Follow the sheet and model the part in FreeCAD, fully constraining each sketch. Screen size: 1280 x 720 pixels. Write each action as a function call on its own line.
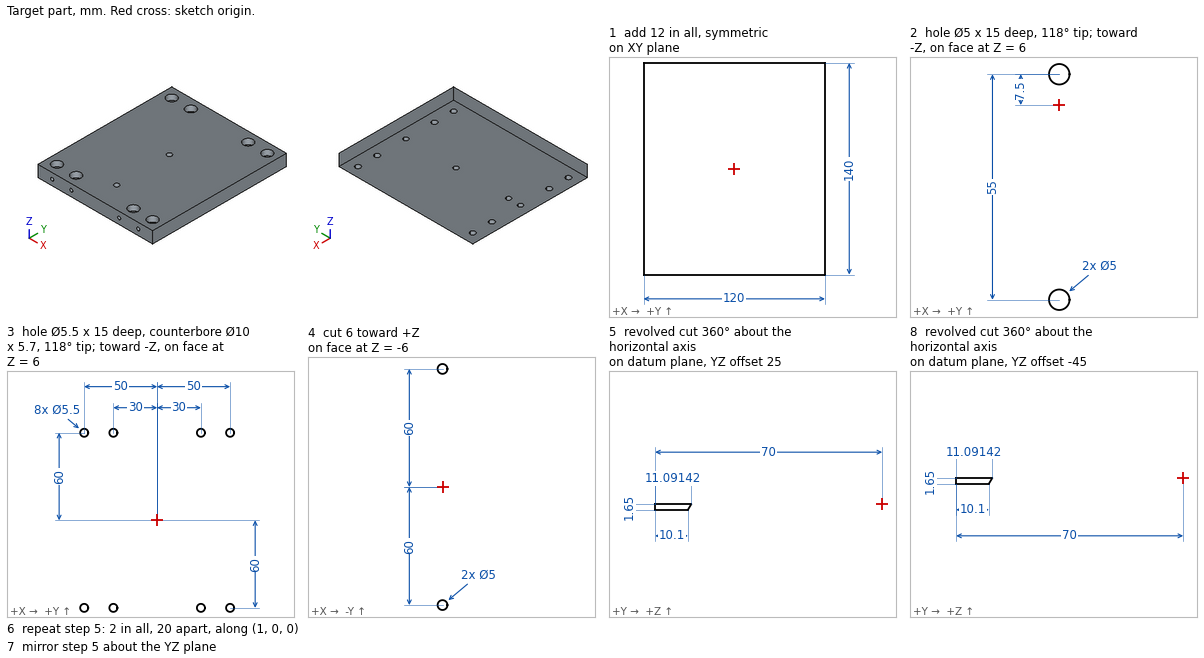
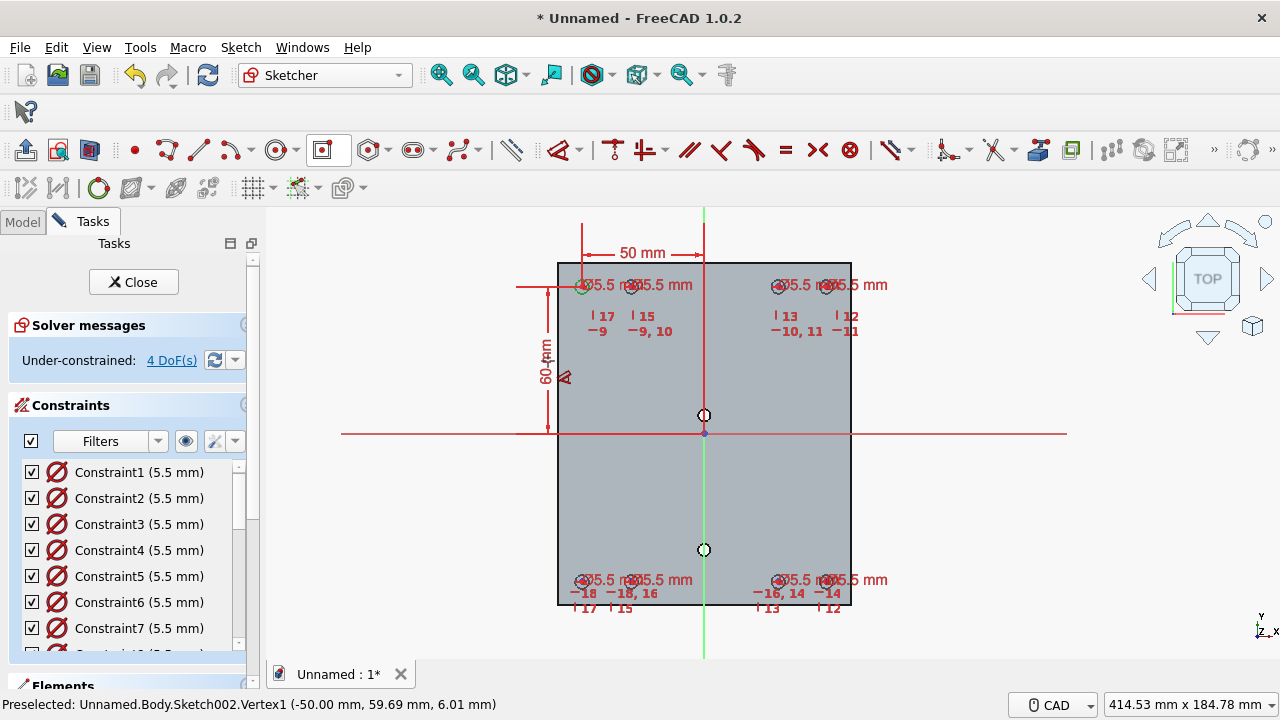
click(631, 287)
click(668, 468)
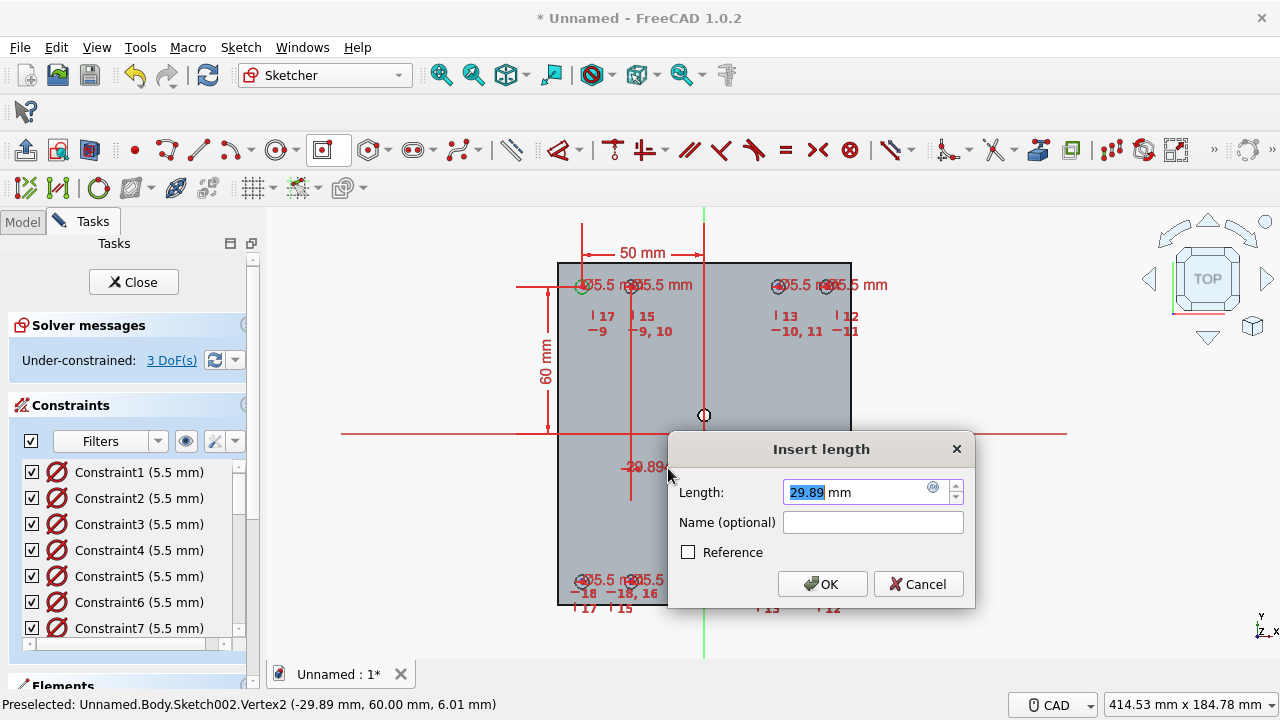
text(30)
key(Return)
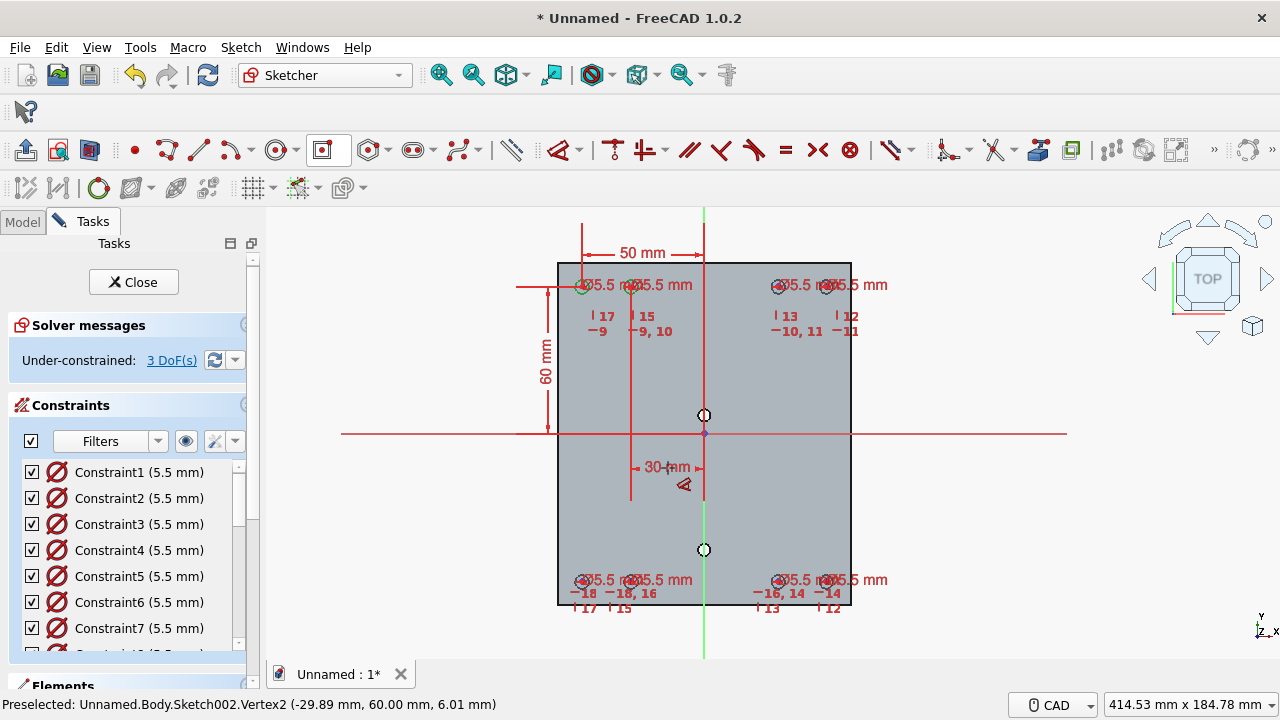
click(778, 287)
click(741, 253)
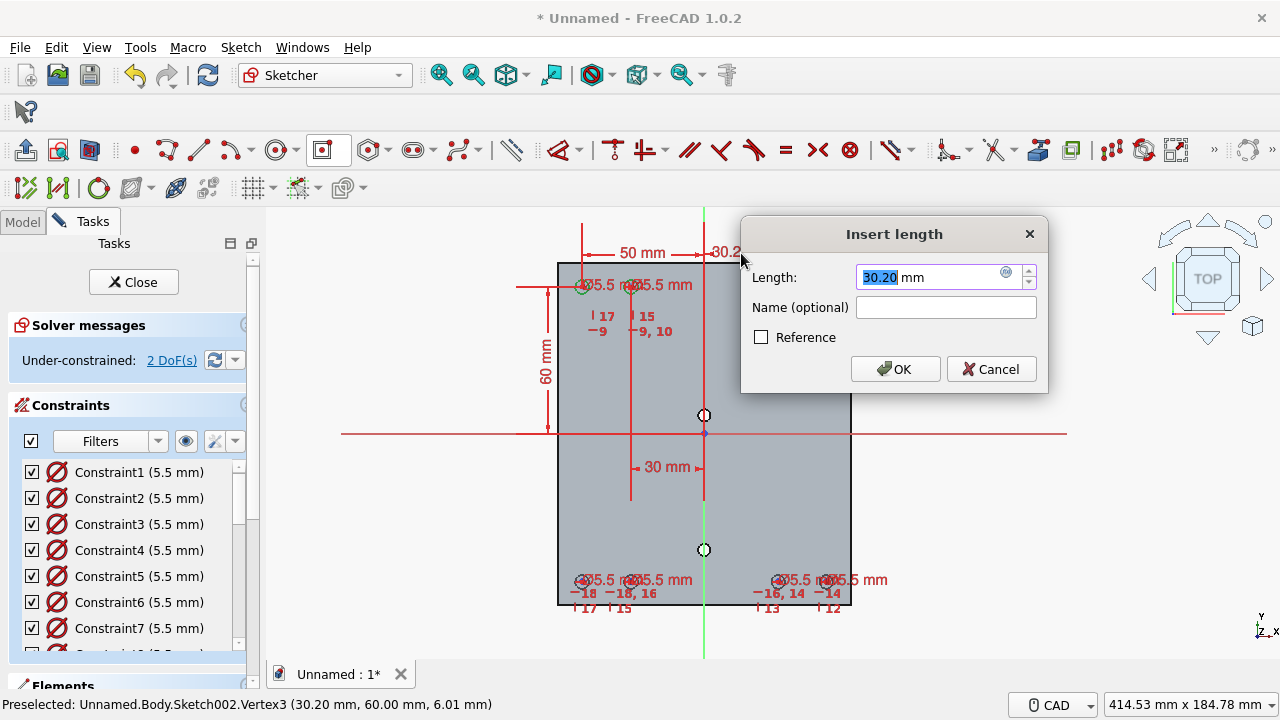
text(30)
key(Return)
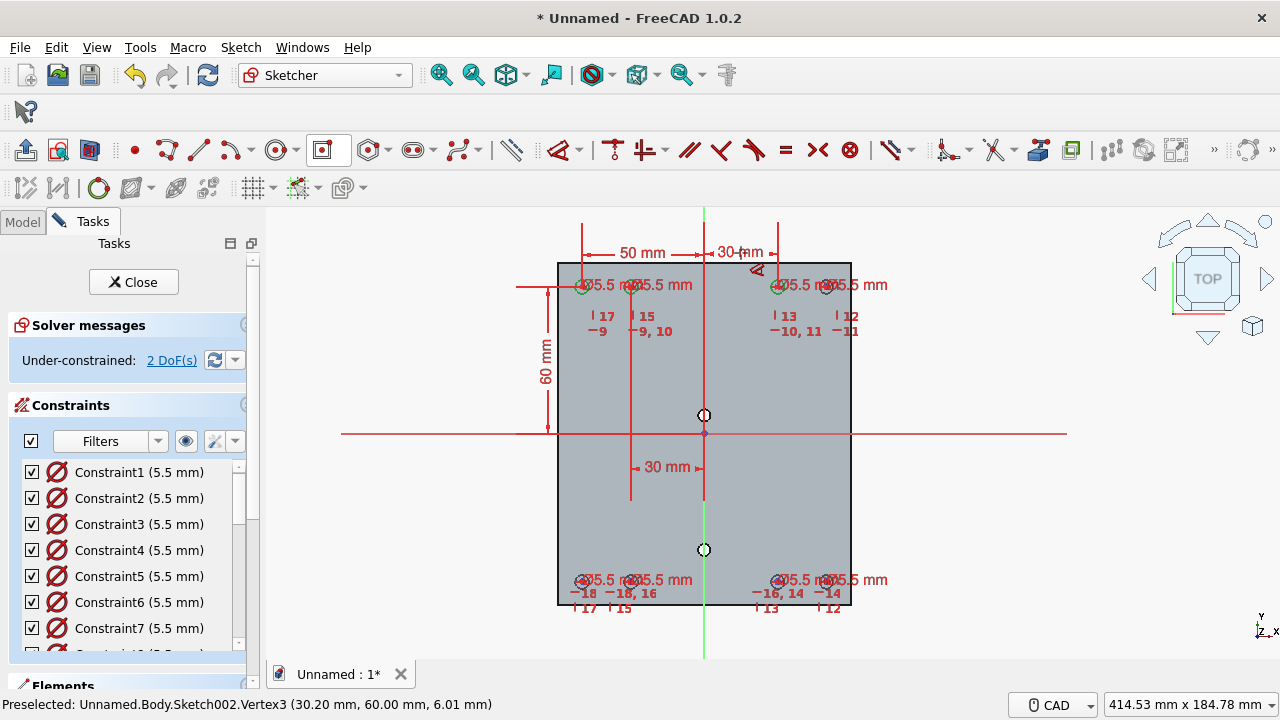
click(826, 287)
click(765, 468)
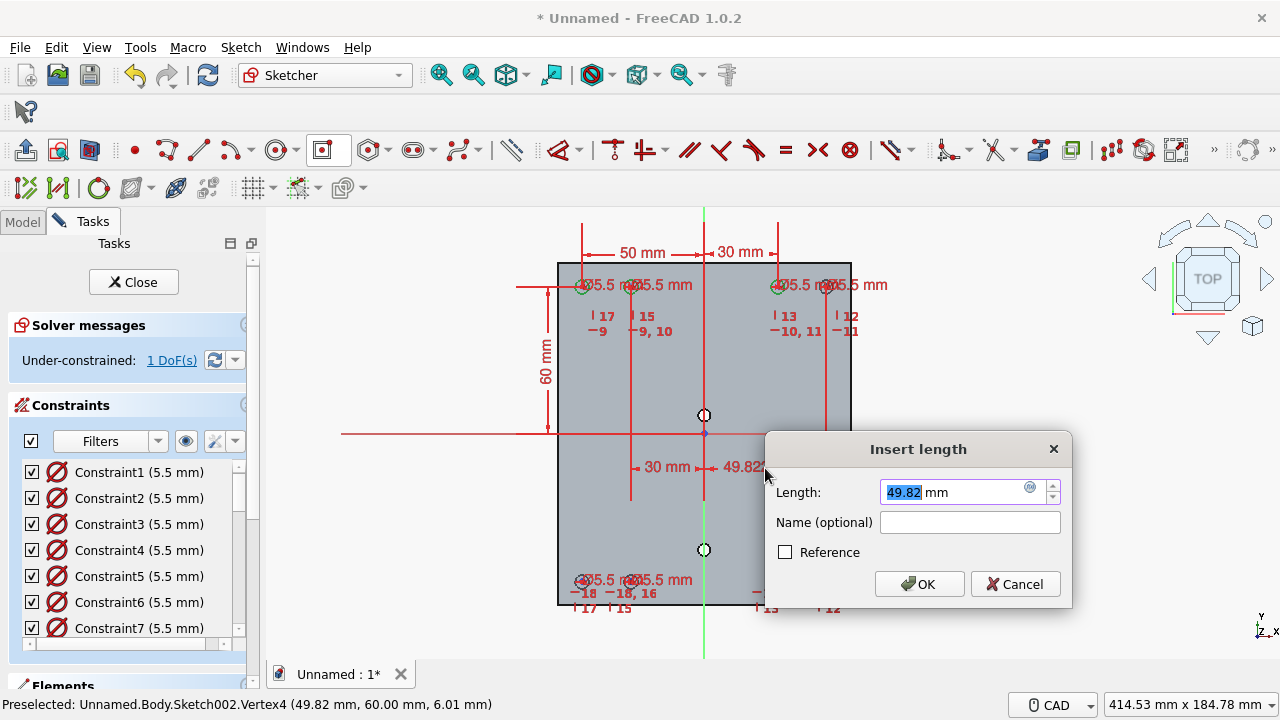
text(50)
key(Return)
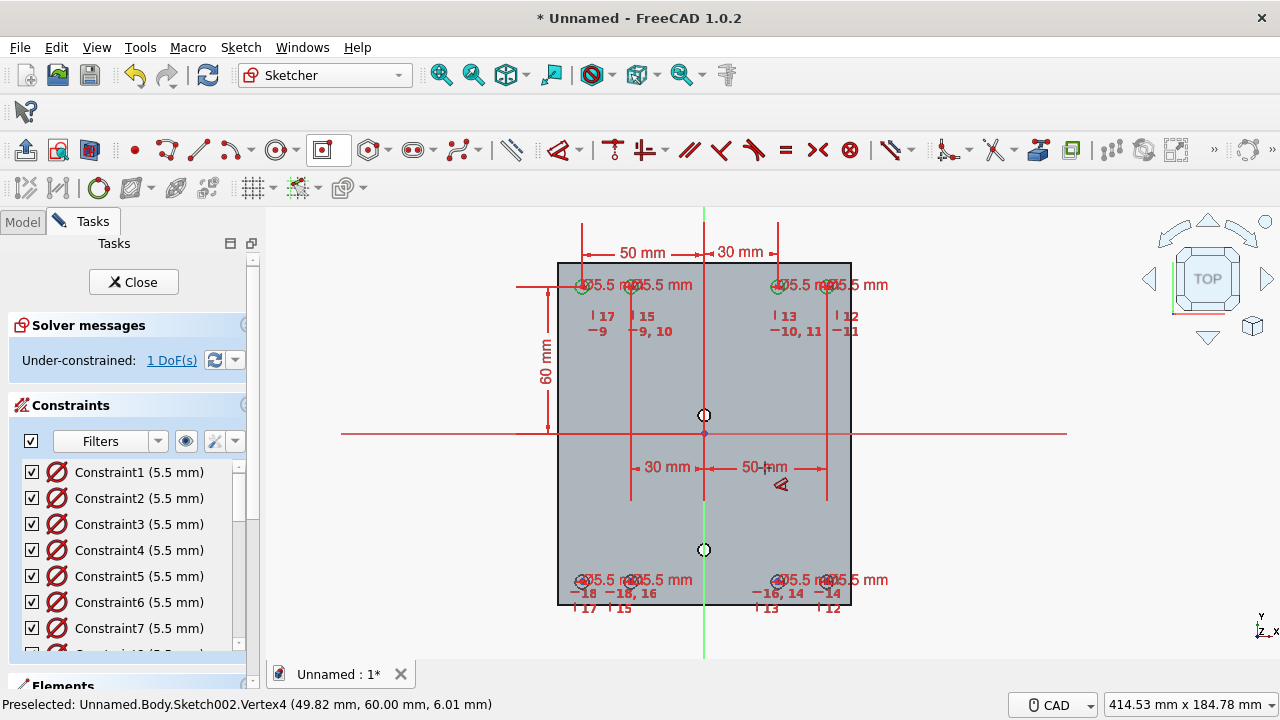
click(827, 582)
click(861, 508)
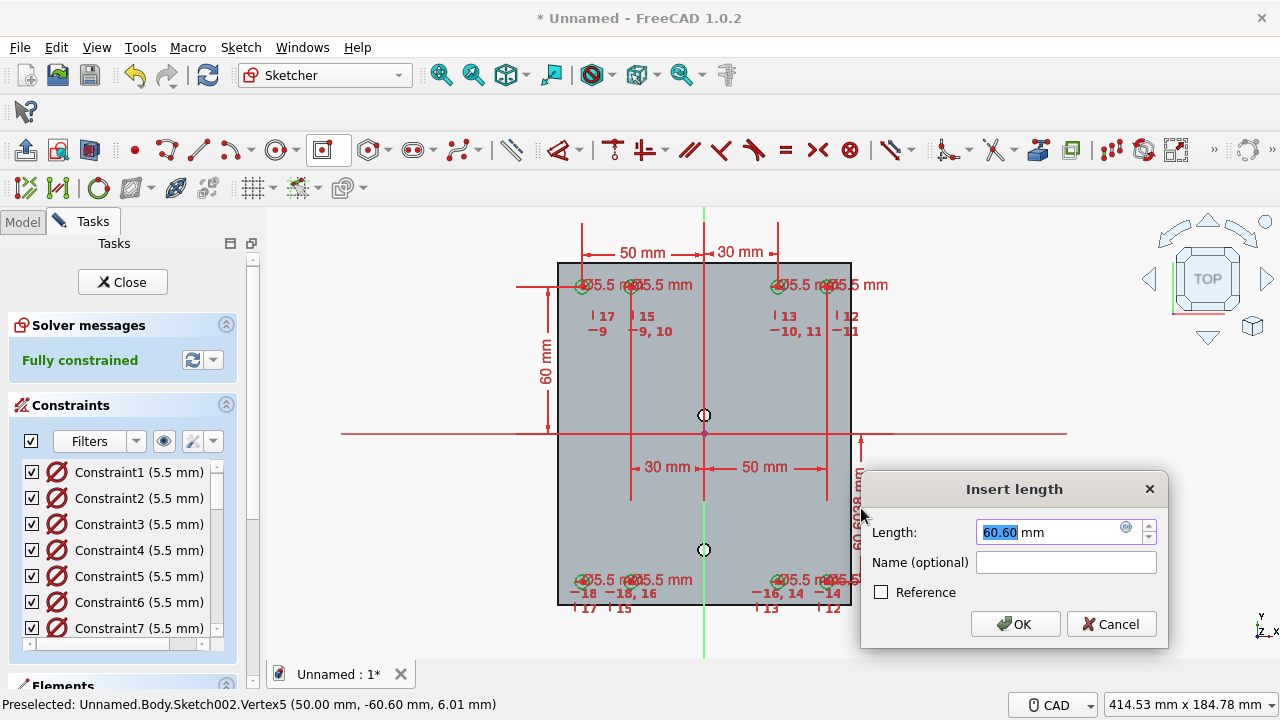
text(60)
key(Return)
key(Escape)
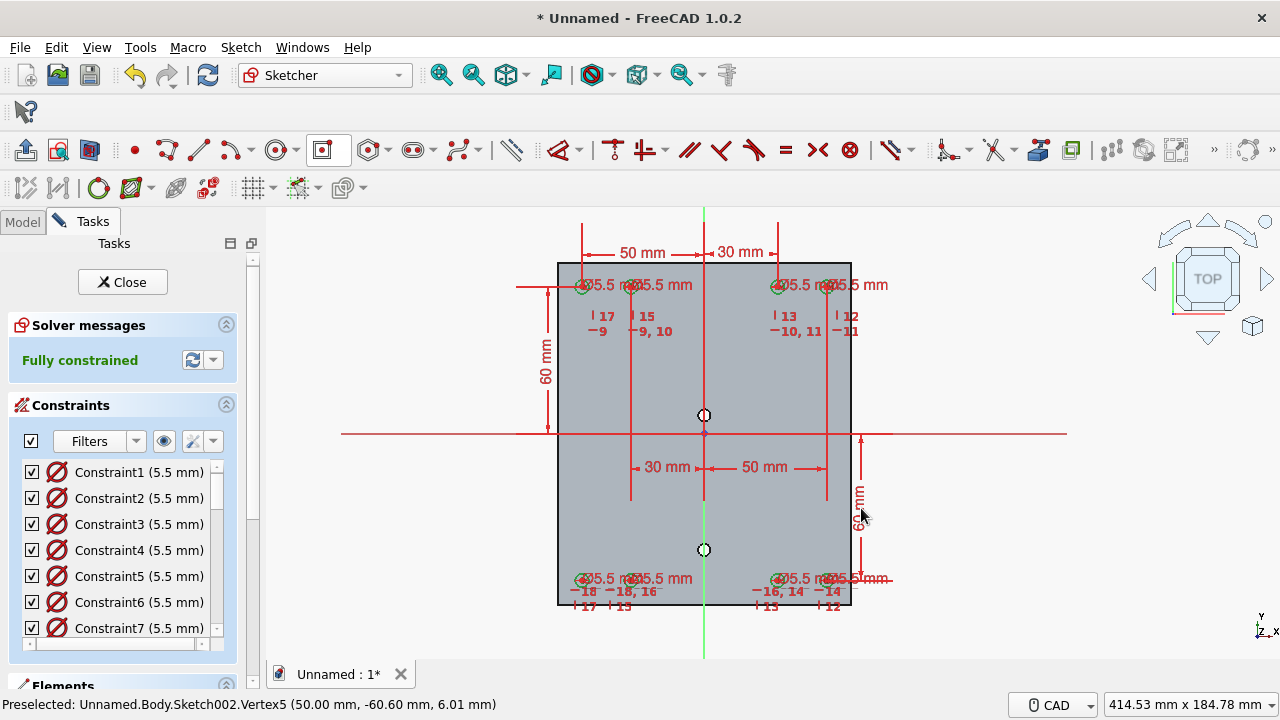
click(123, 282)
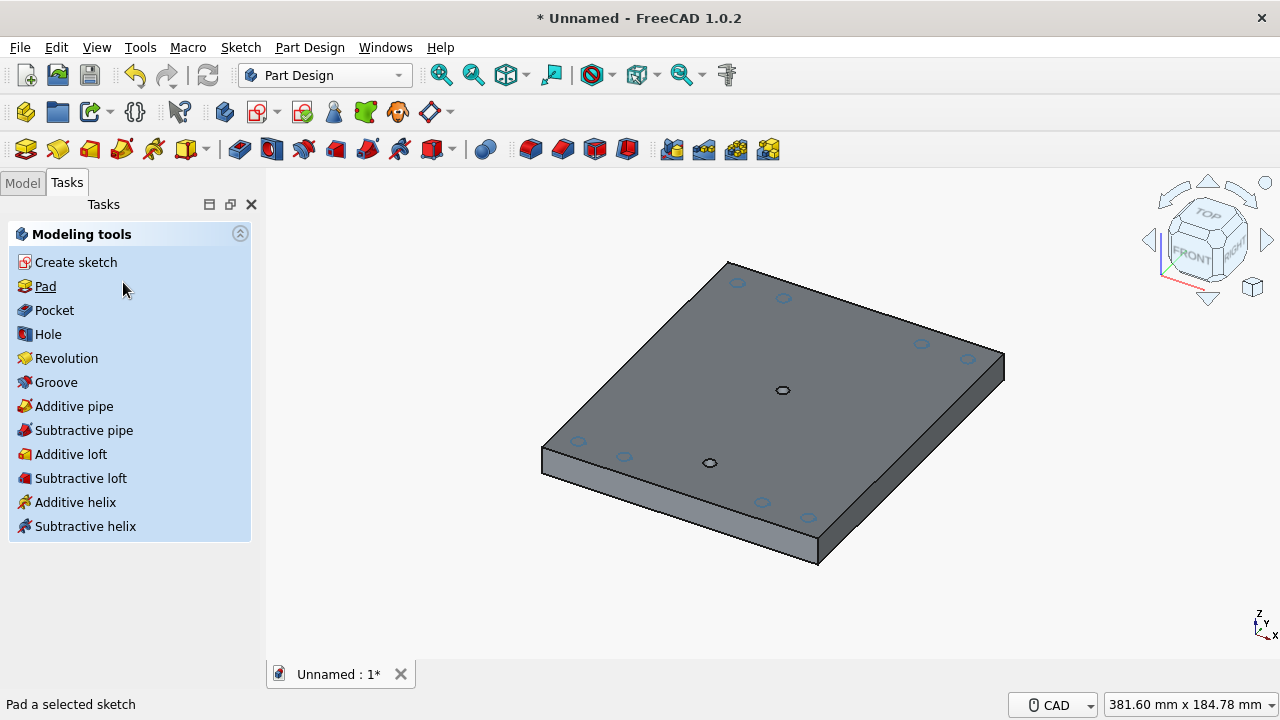
click(272, 150)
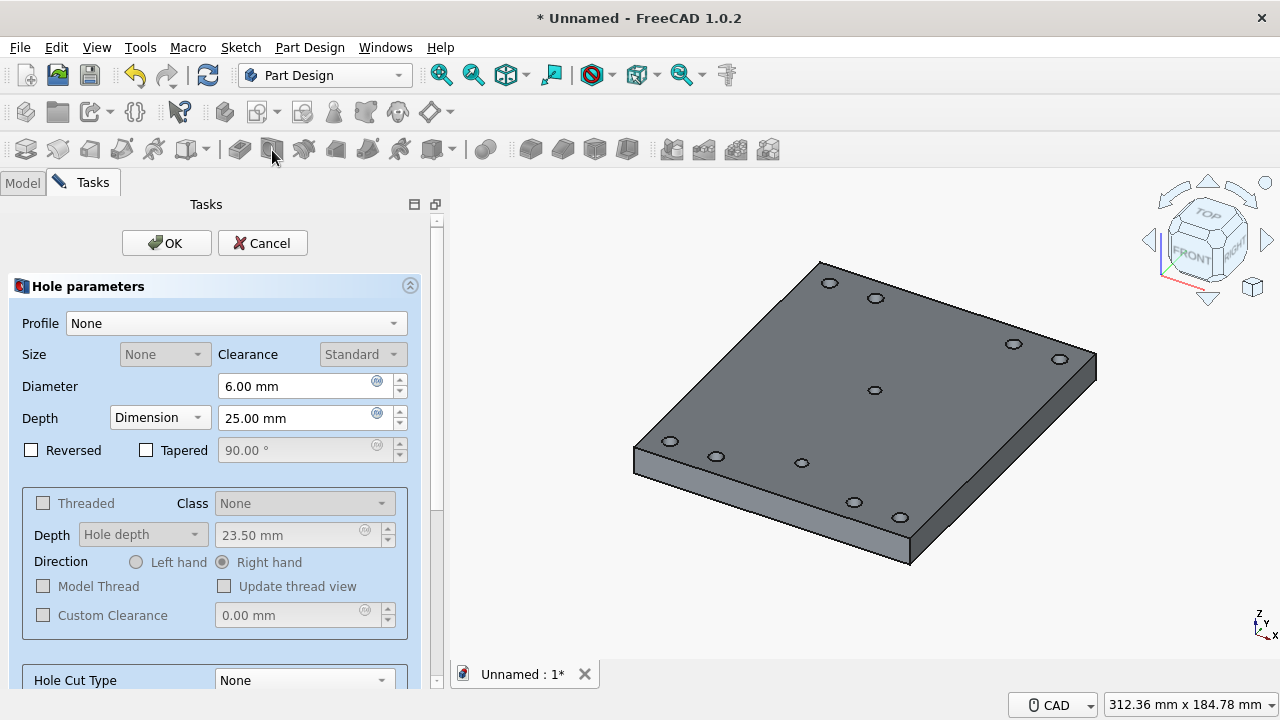
triple_click(305, 386)